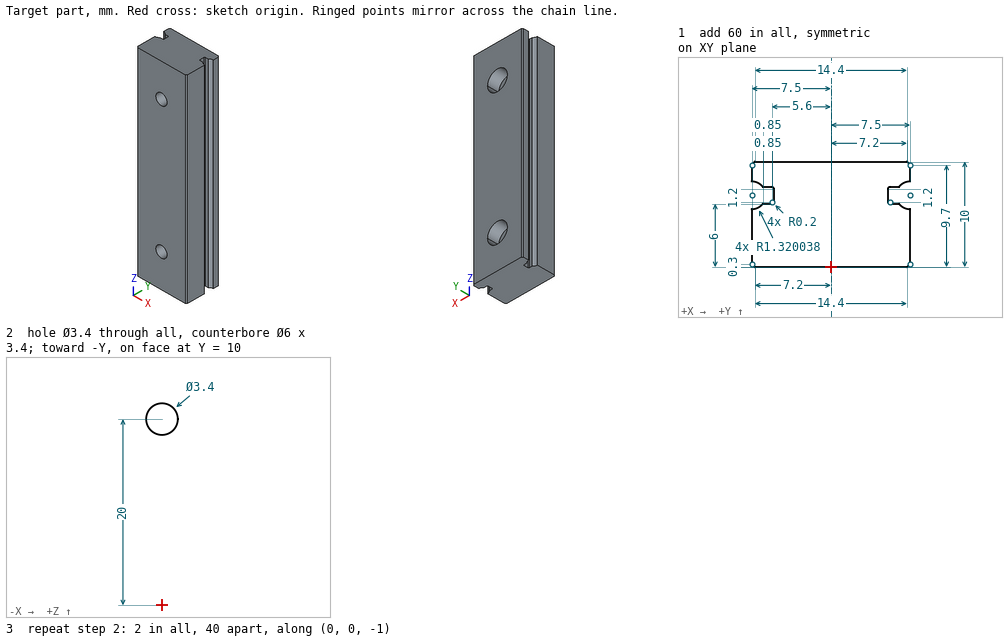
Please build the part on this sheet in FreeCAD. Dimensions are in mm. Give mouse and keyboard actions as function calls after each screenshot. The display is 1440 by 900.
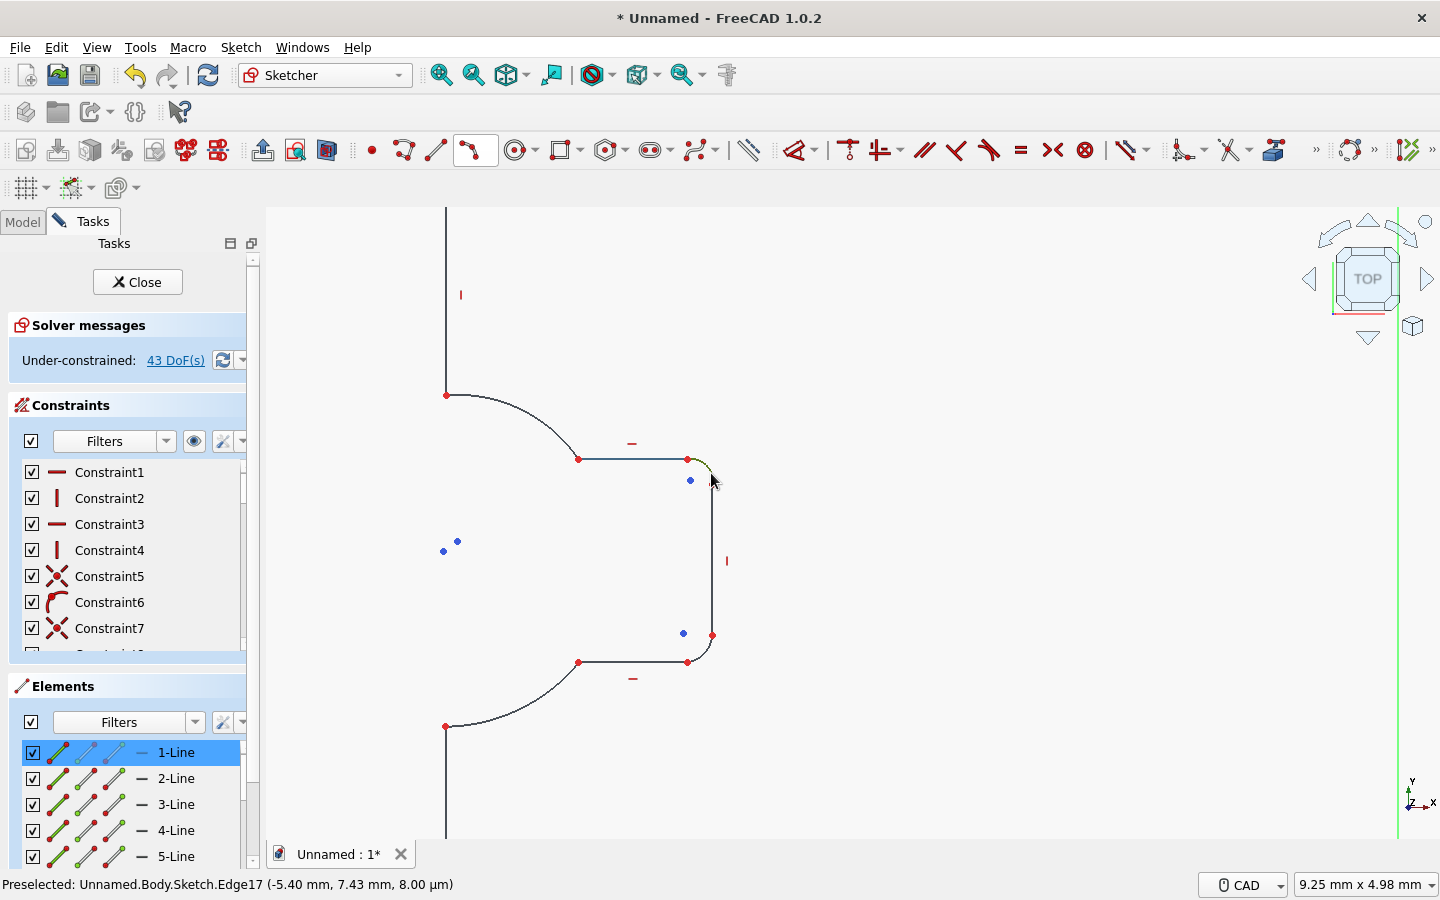
click(990, 150)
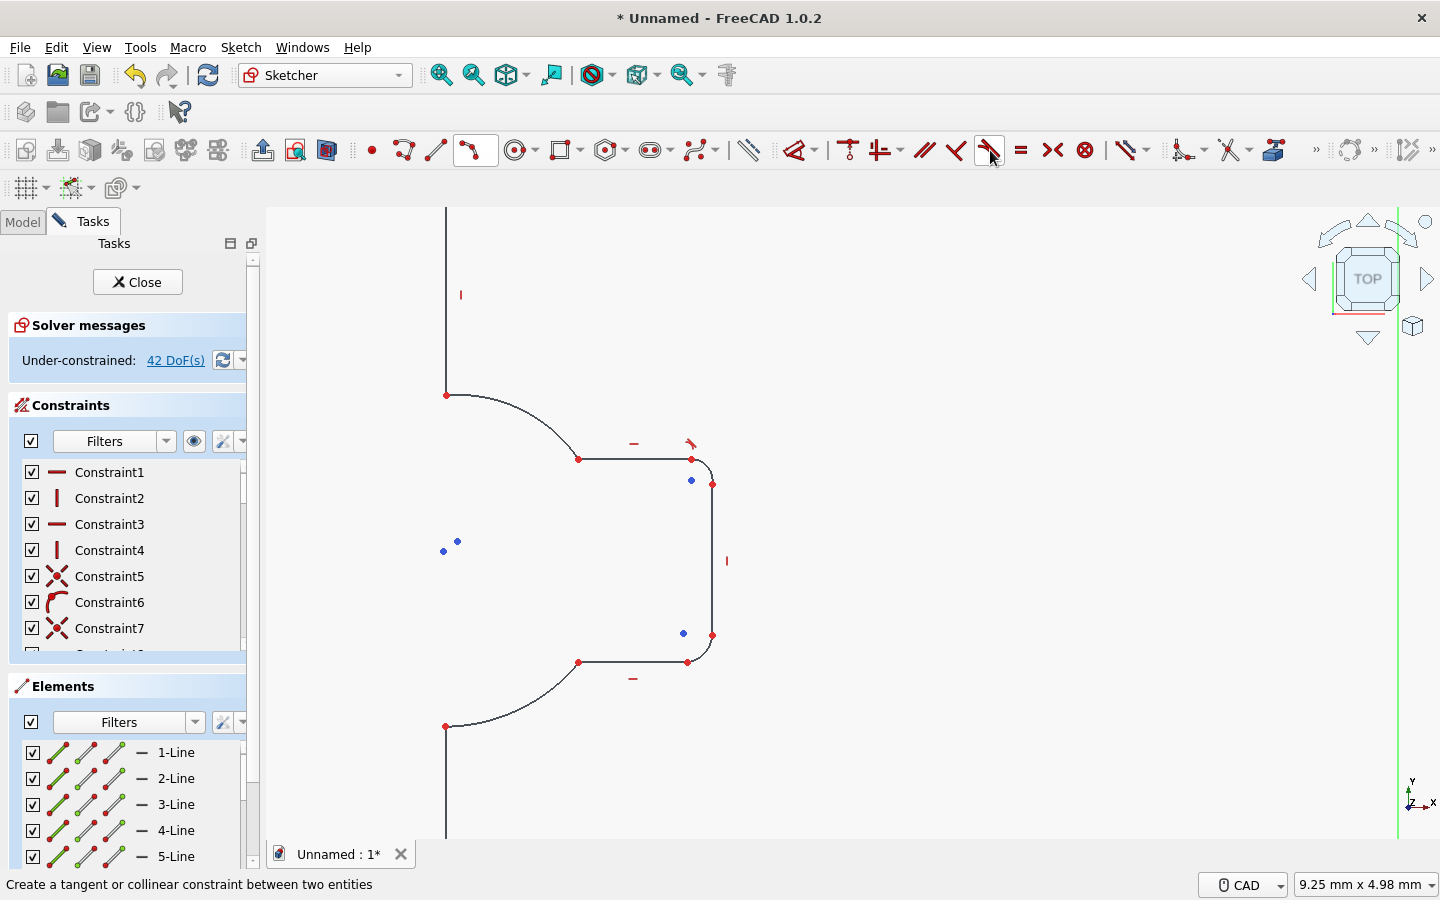
click(712, 530)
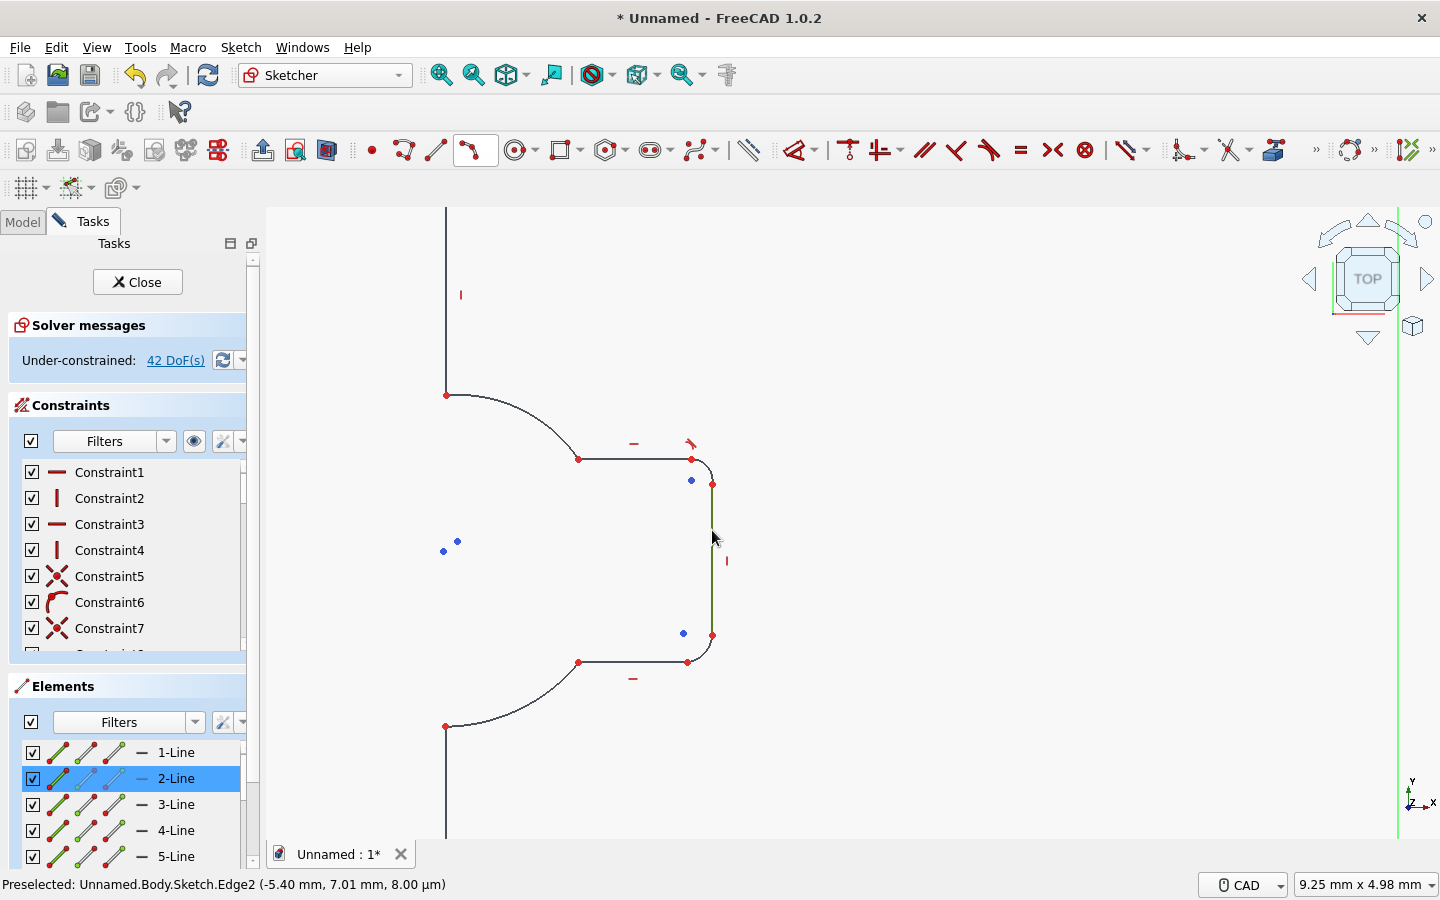
scroll(711, 474, up, 2)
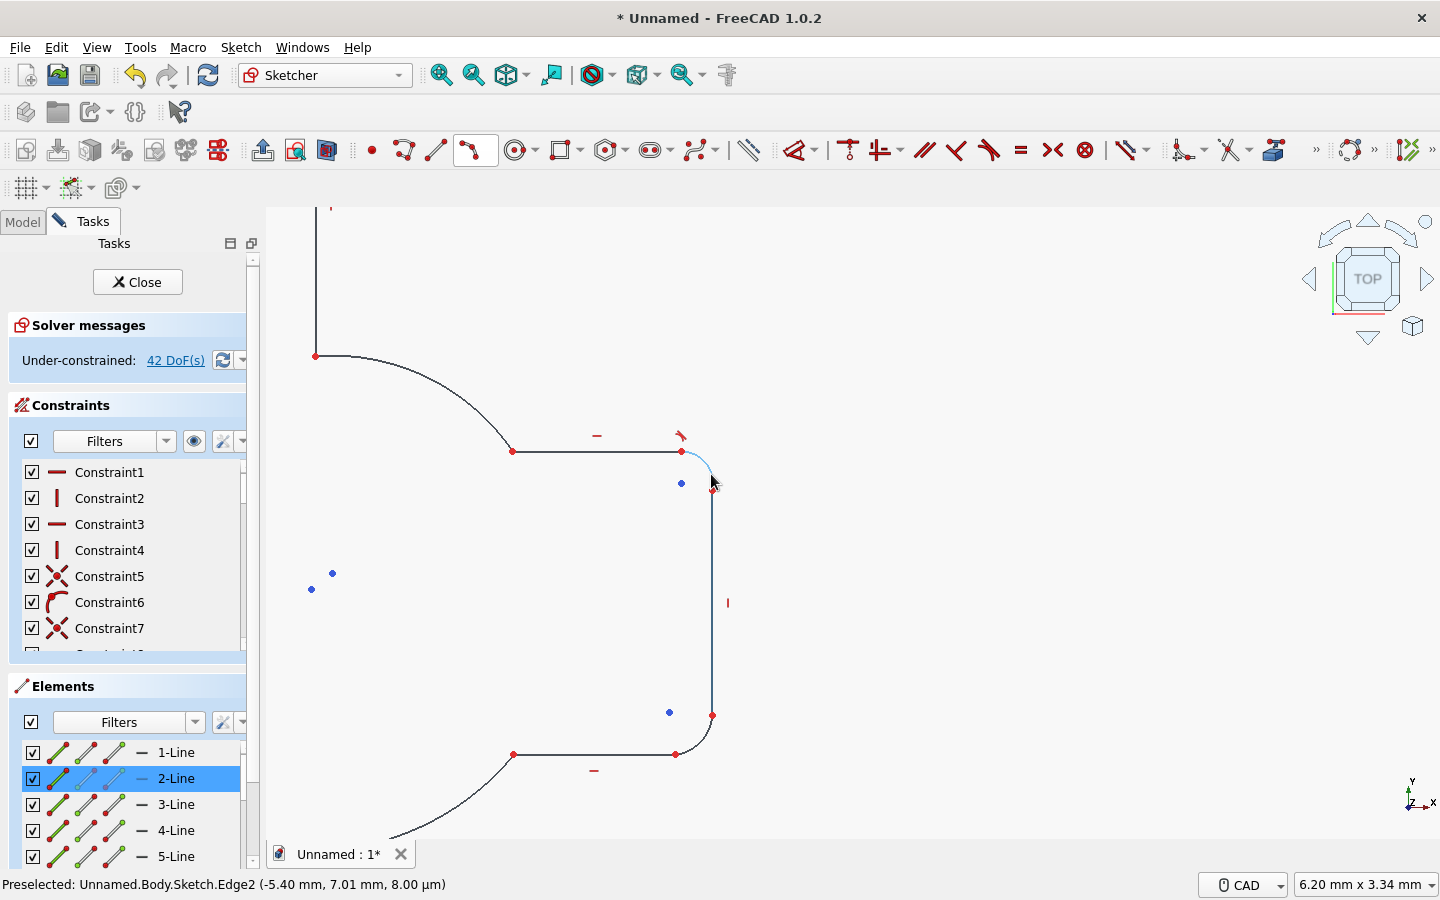
click(711, 473)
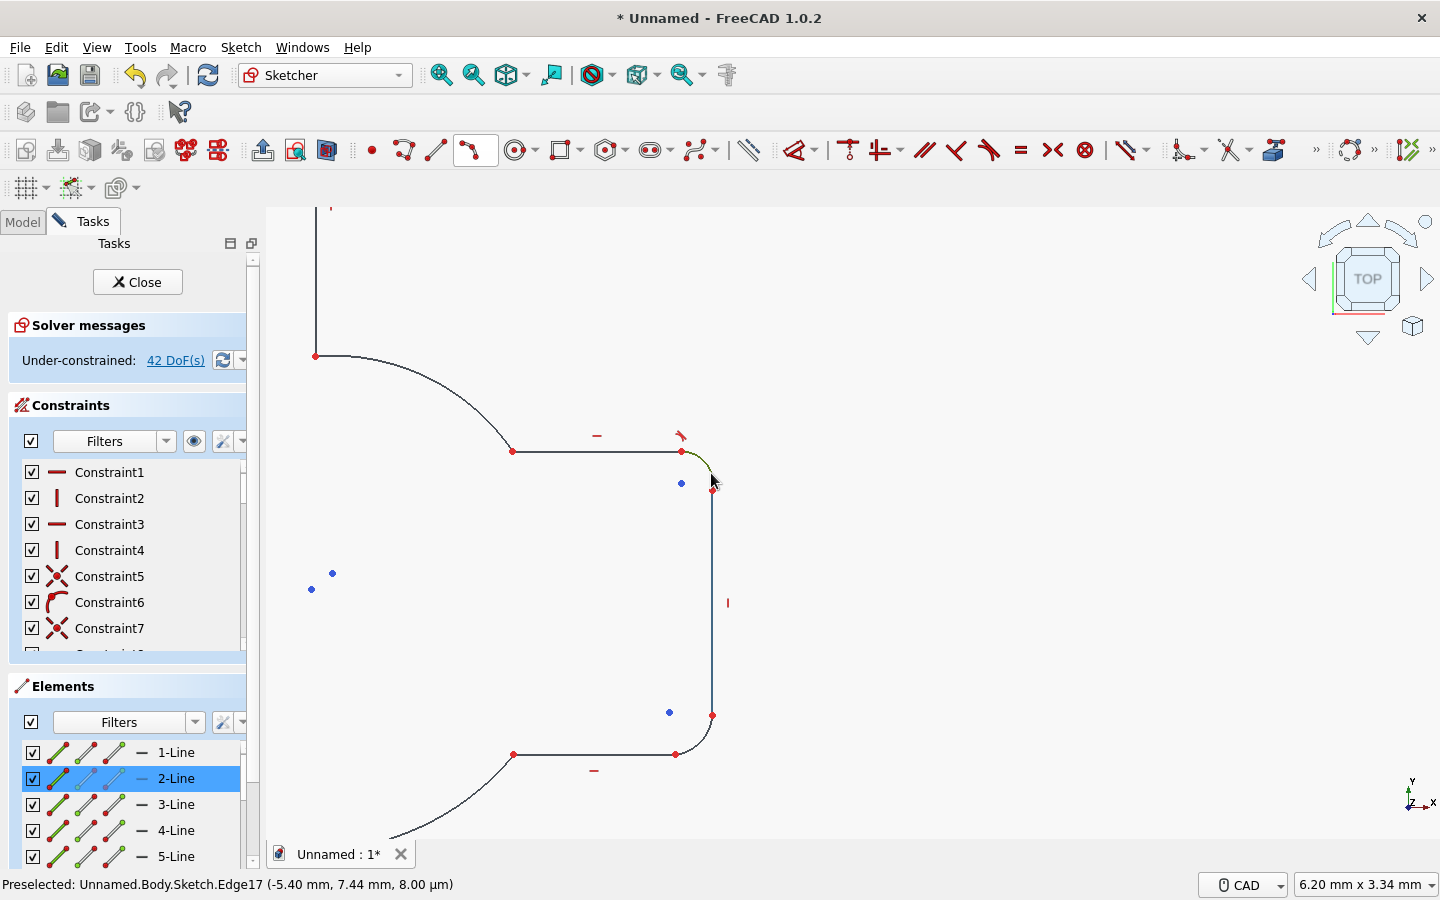
click(990, 150)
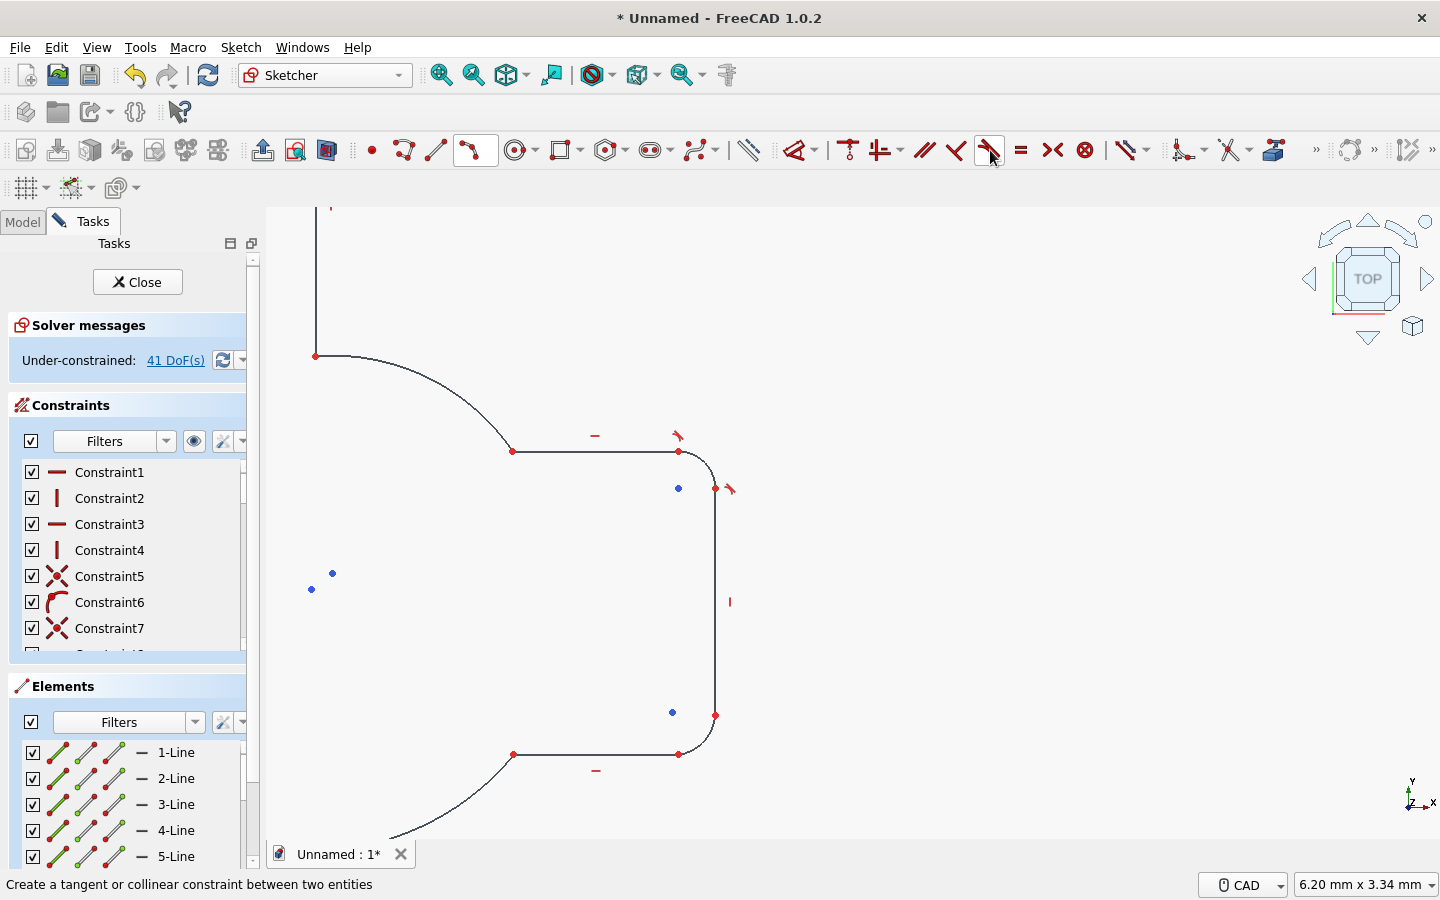
scroll(544, 418, down, 8)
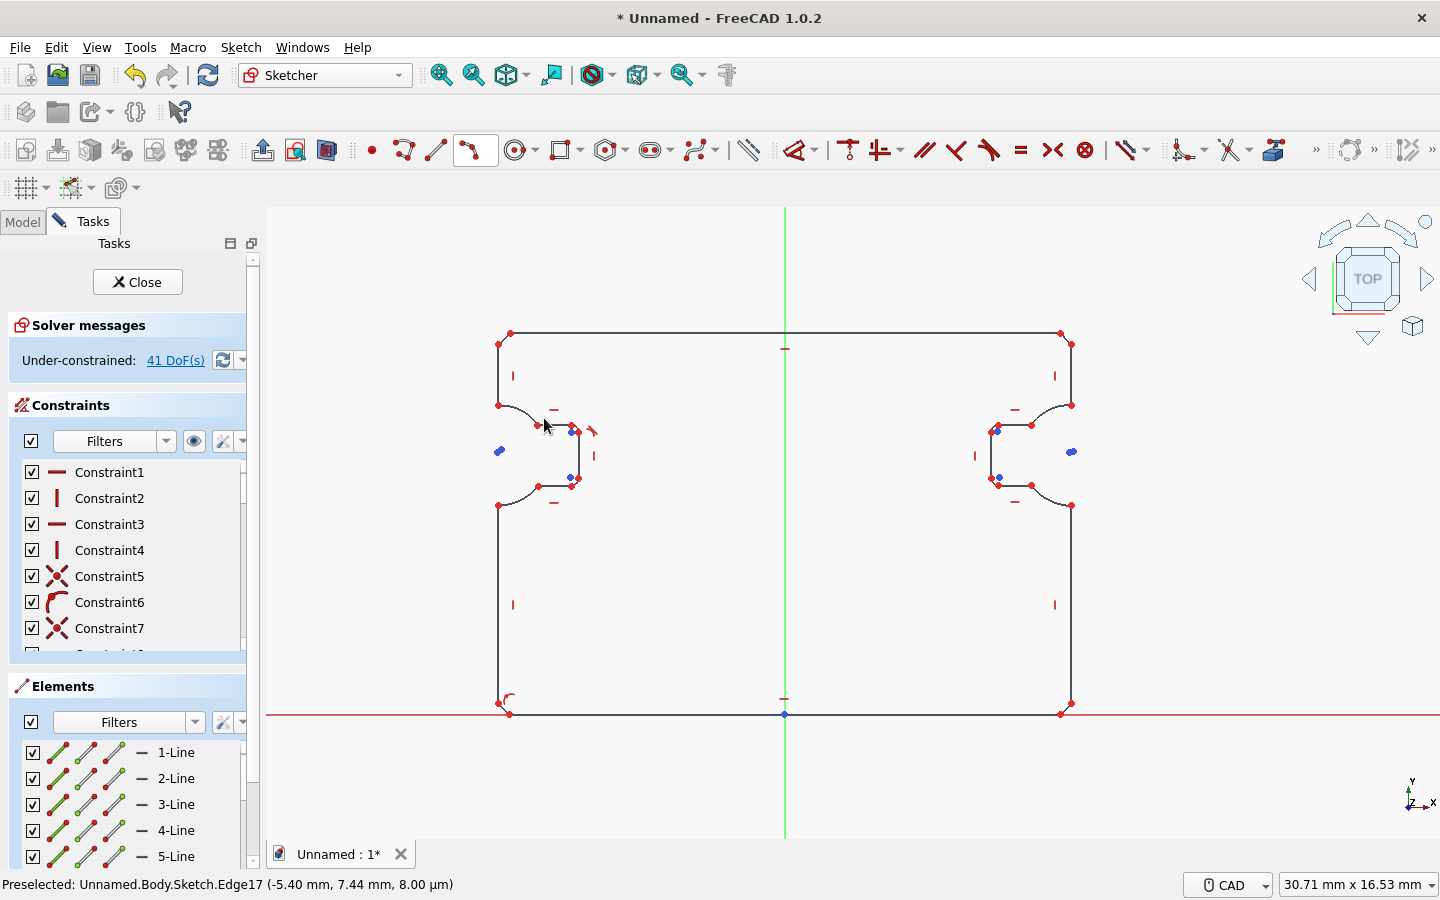
click(579, 446)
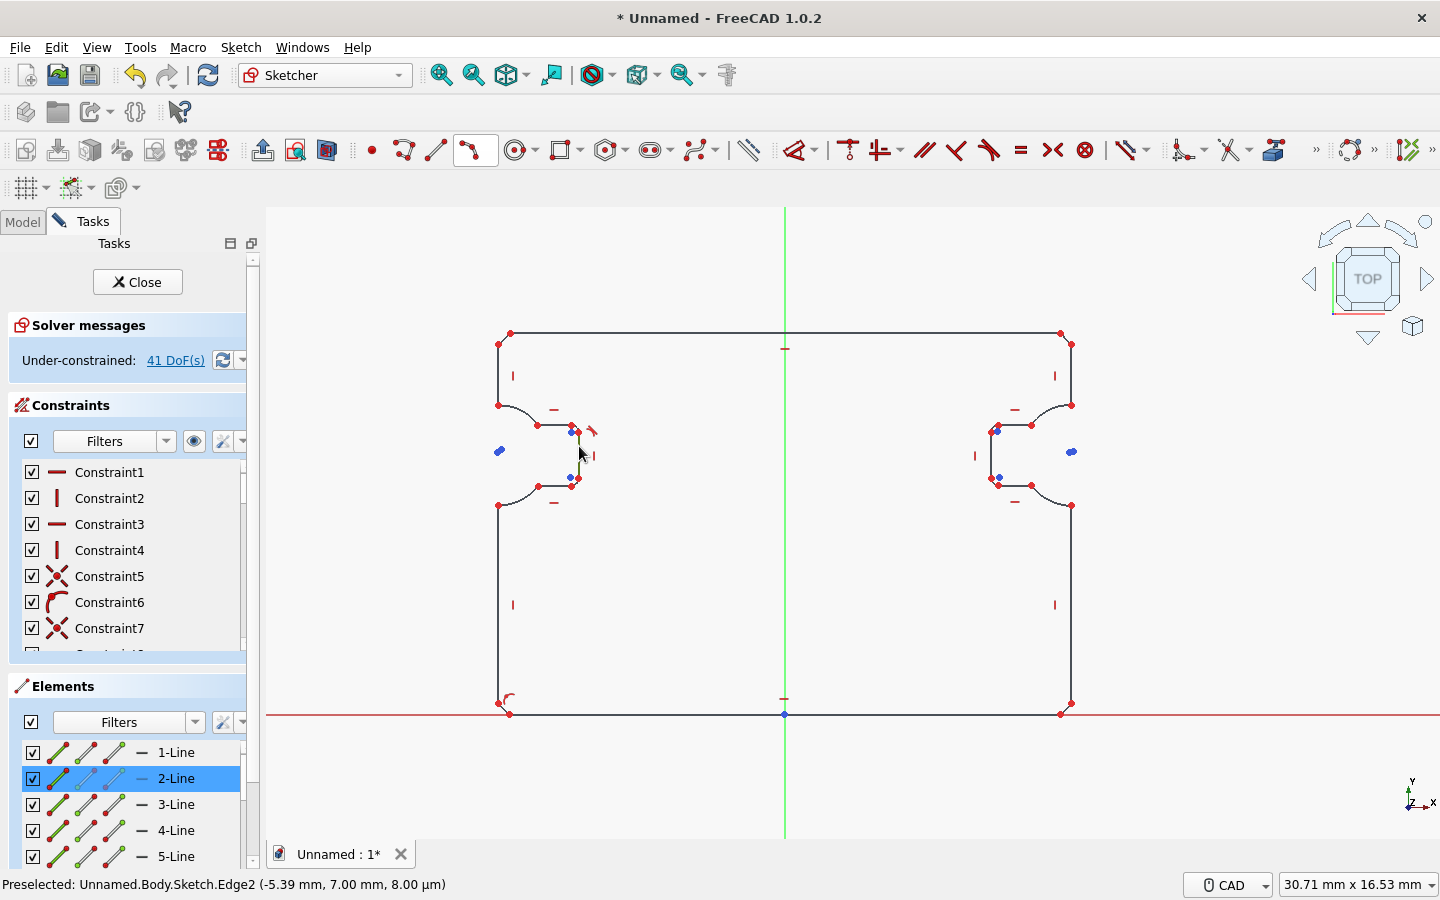
scroll(576, 484, up, 5)